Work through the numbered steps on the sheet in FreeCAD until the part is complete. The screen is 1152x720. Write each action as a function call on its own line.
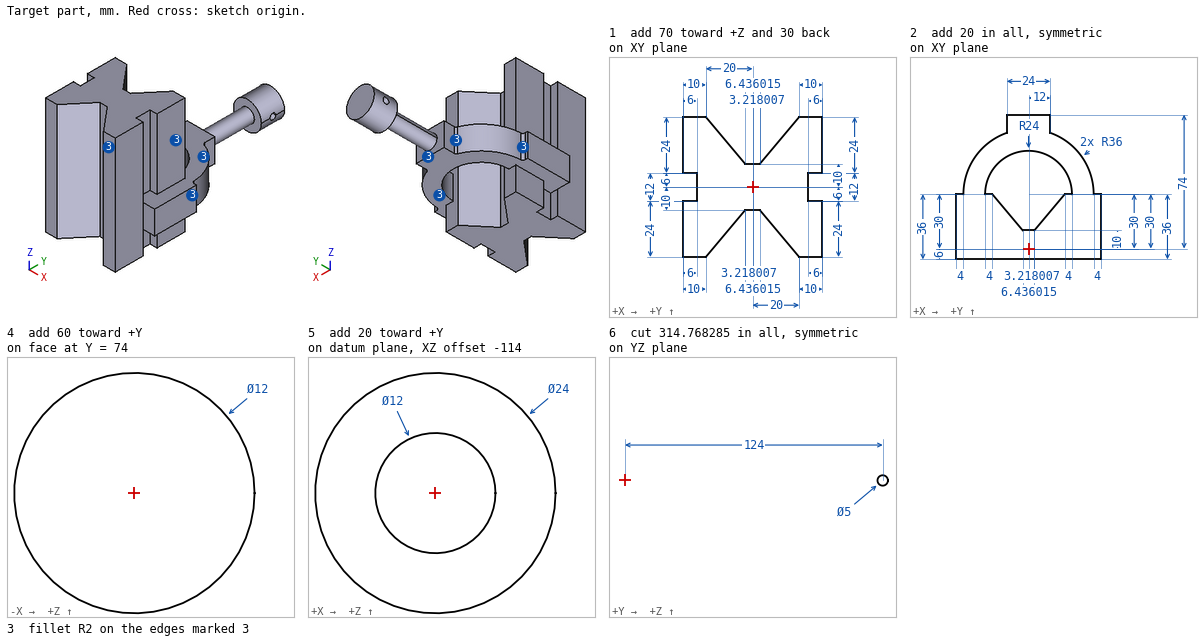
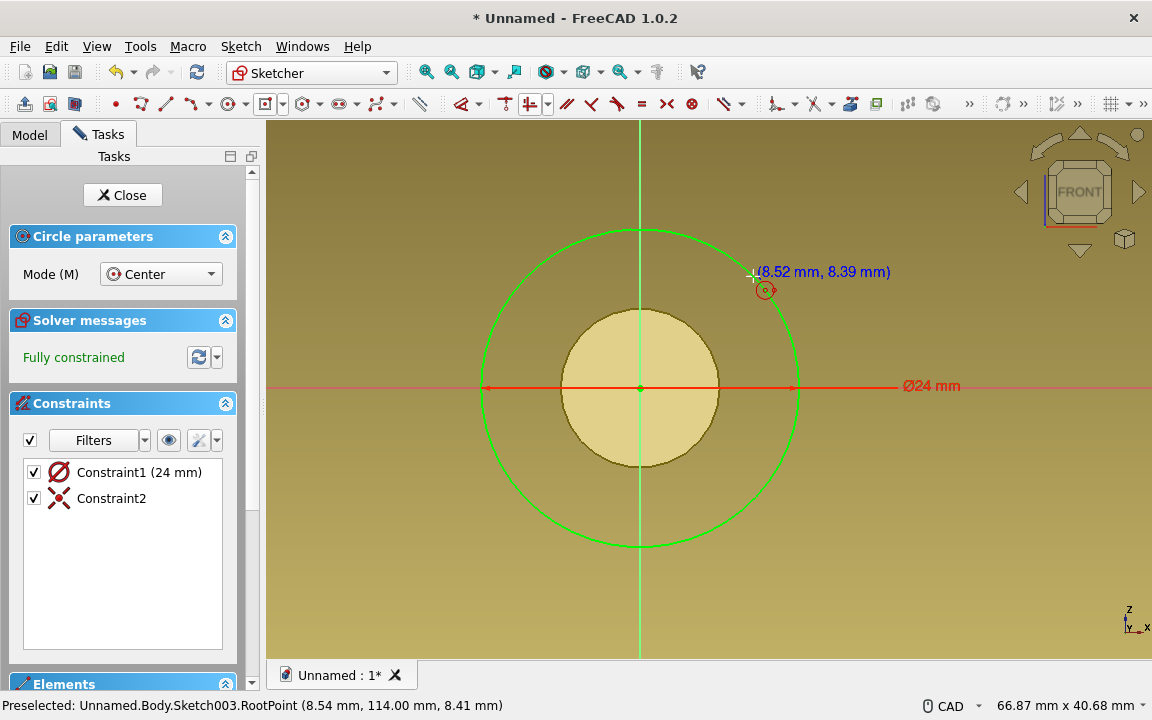
click(640, 388)
move(696, 332)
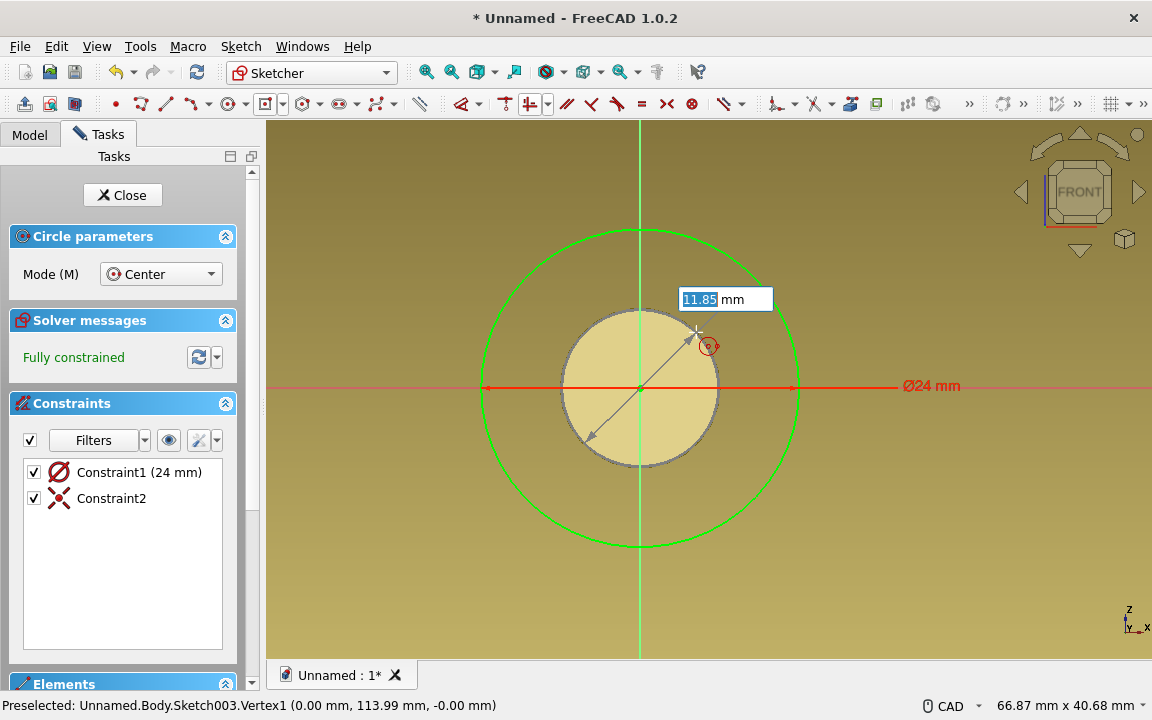
text(12)
key(Return)
key(Escape)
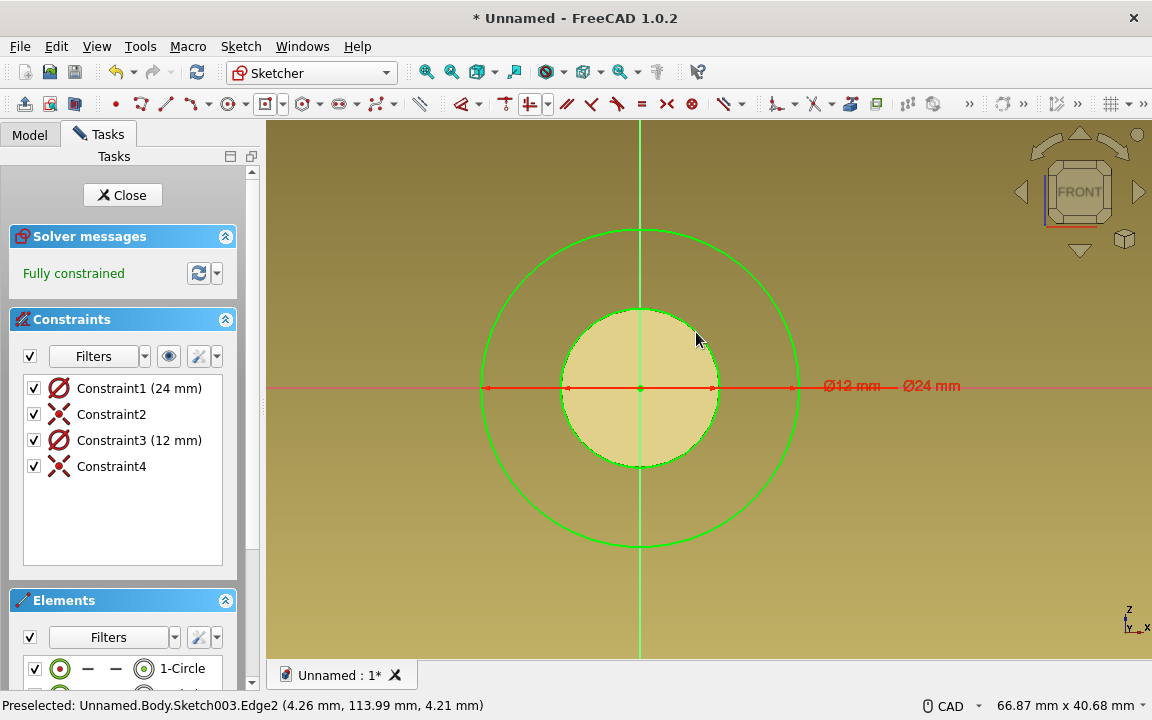
click(123, 195)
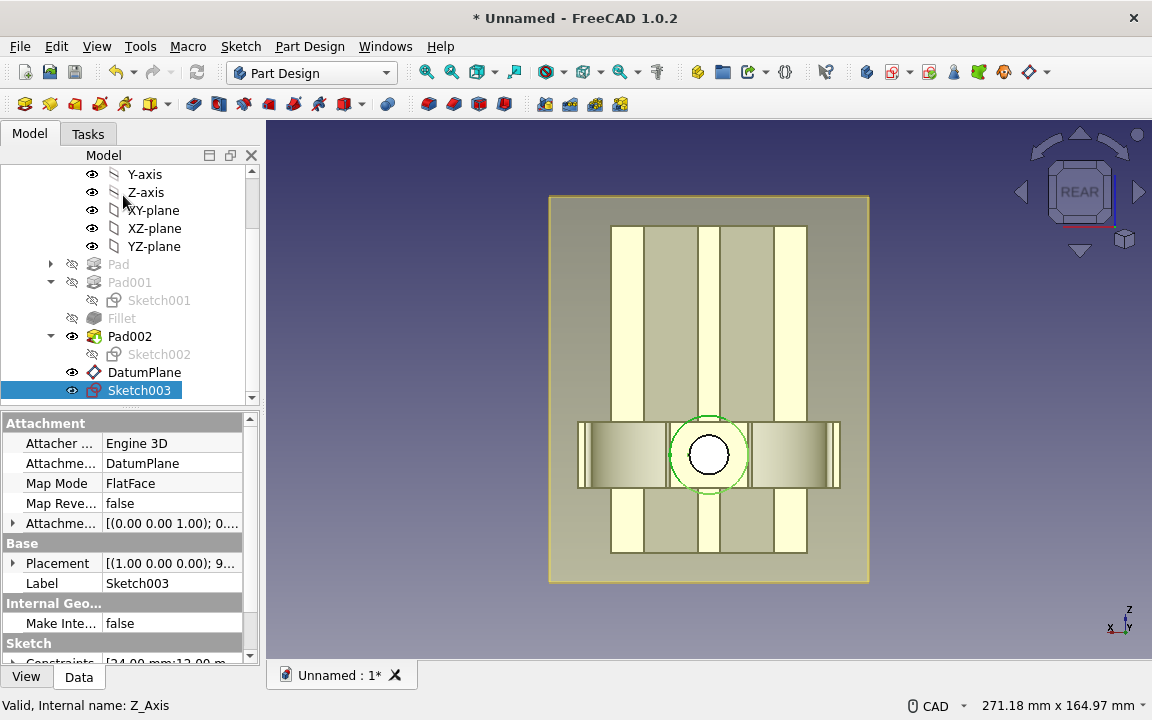
click(25, 104)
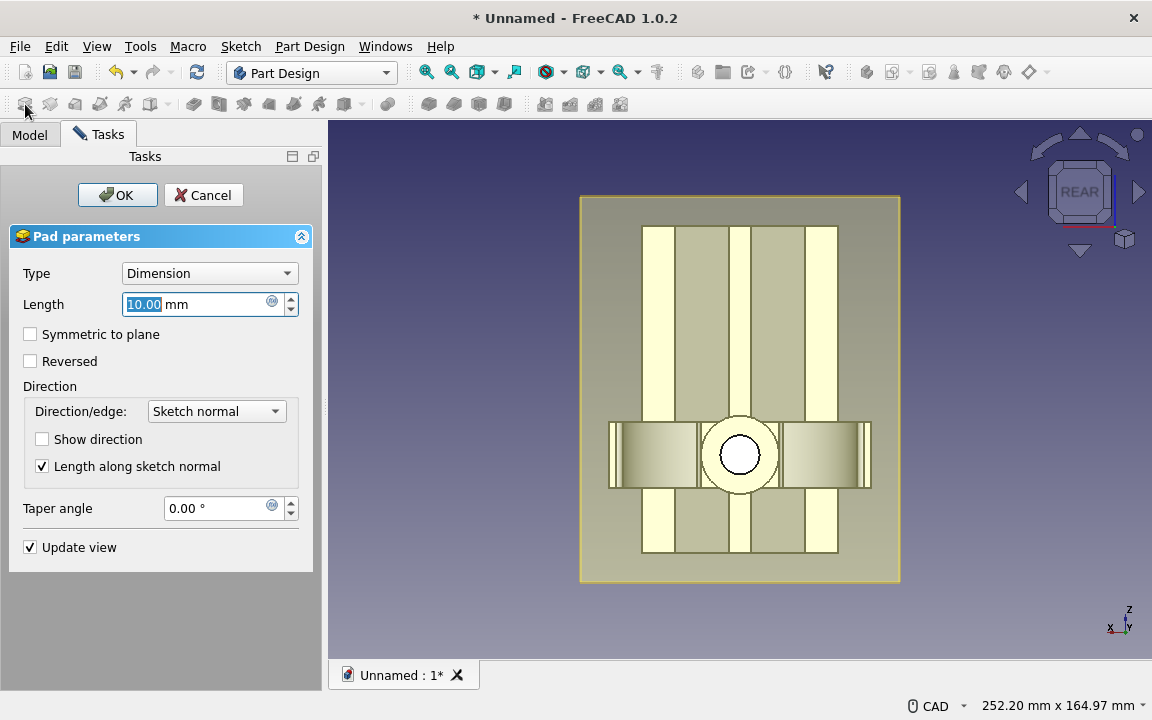
text(20)
key(Tab)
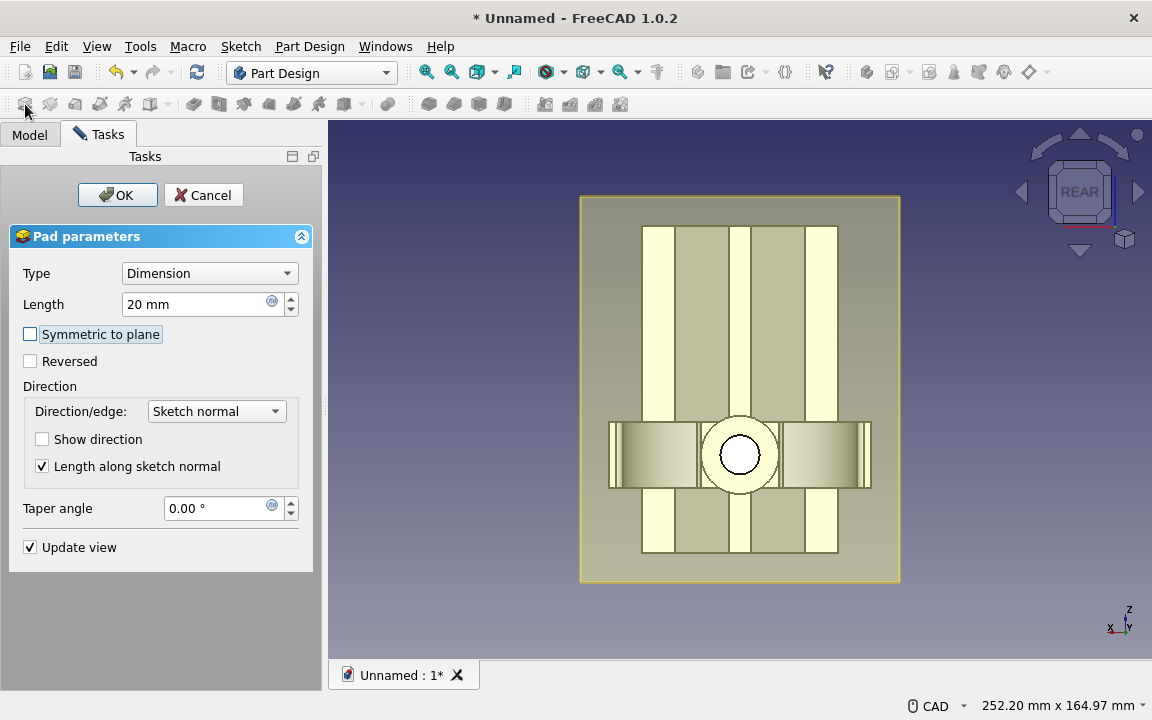
click(31, 361)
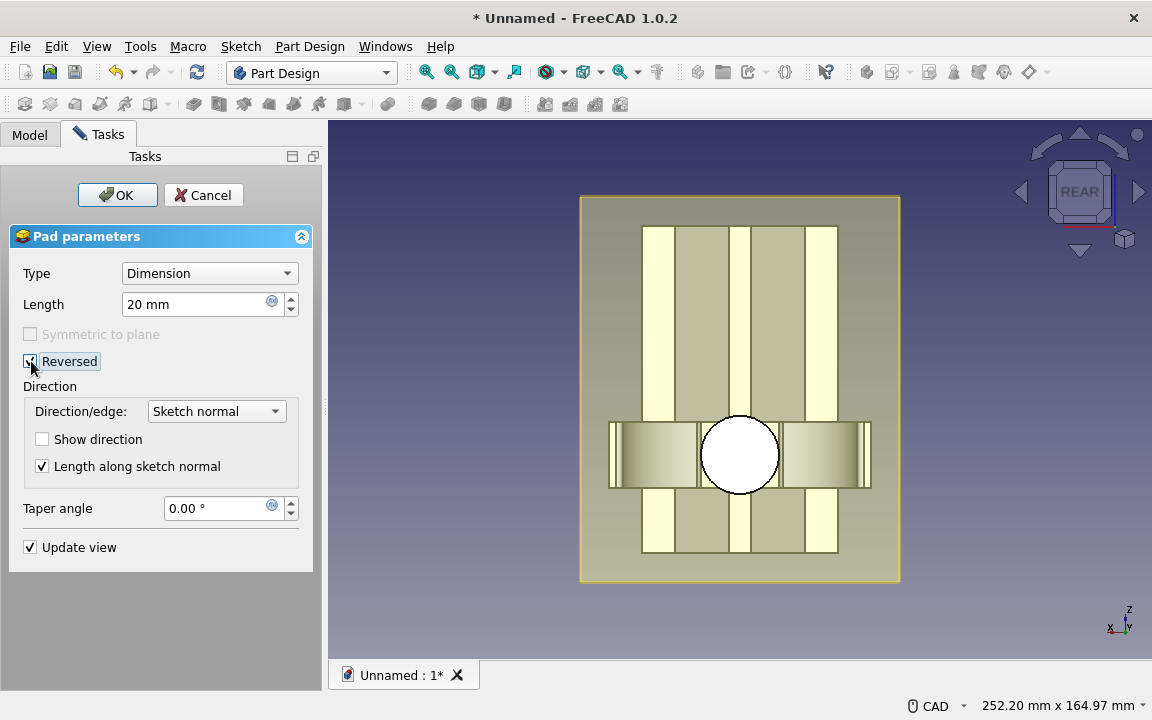
click(118, 195)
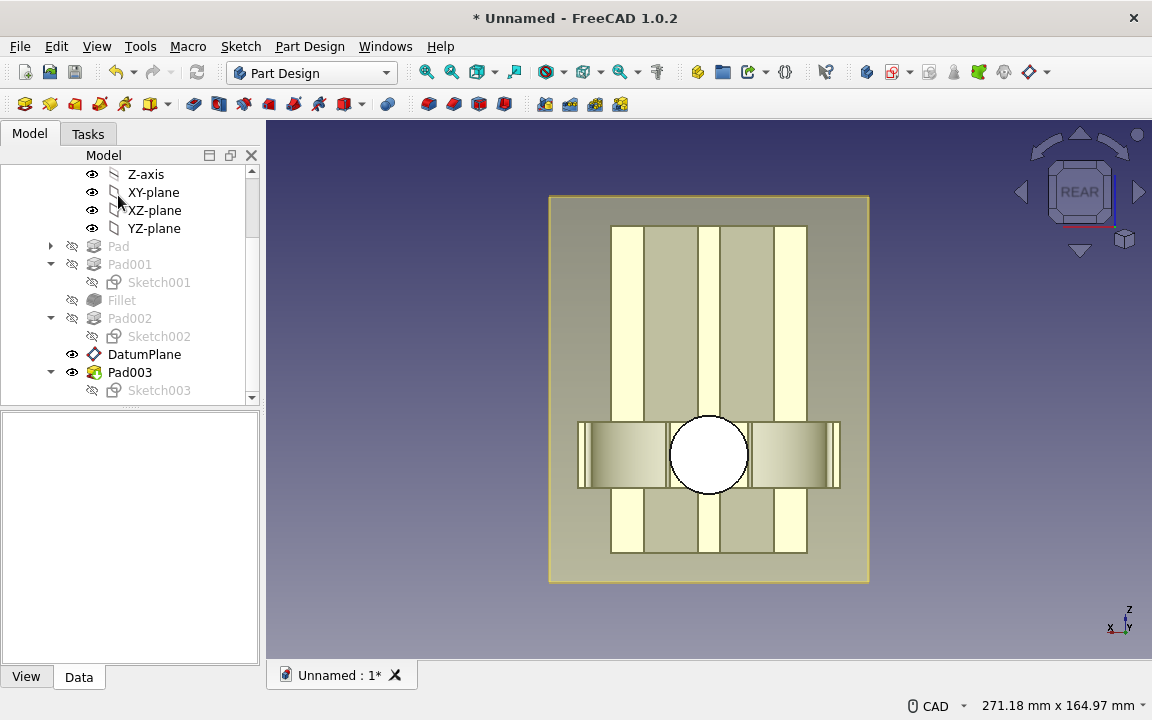
click(117, 354)
key(space)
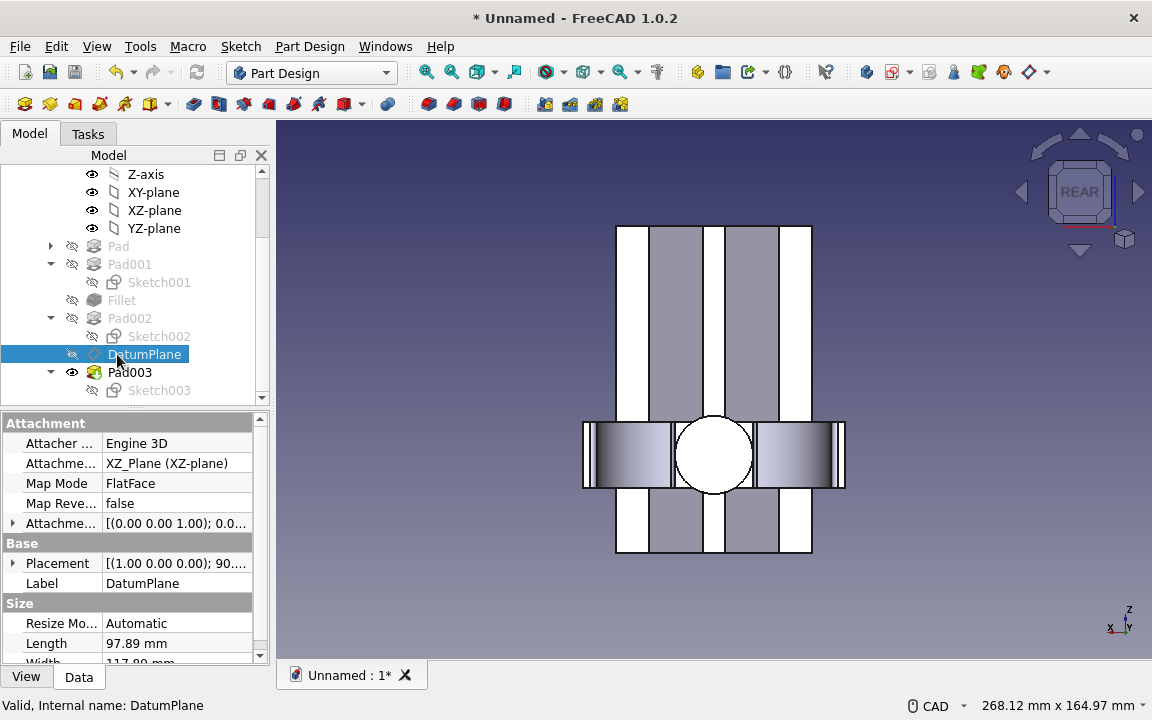
click(316, 619)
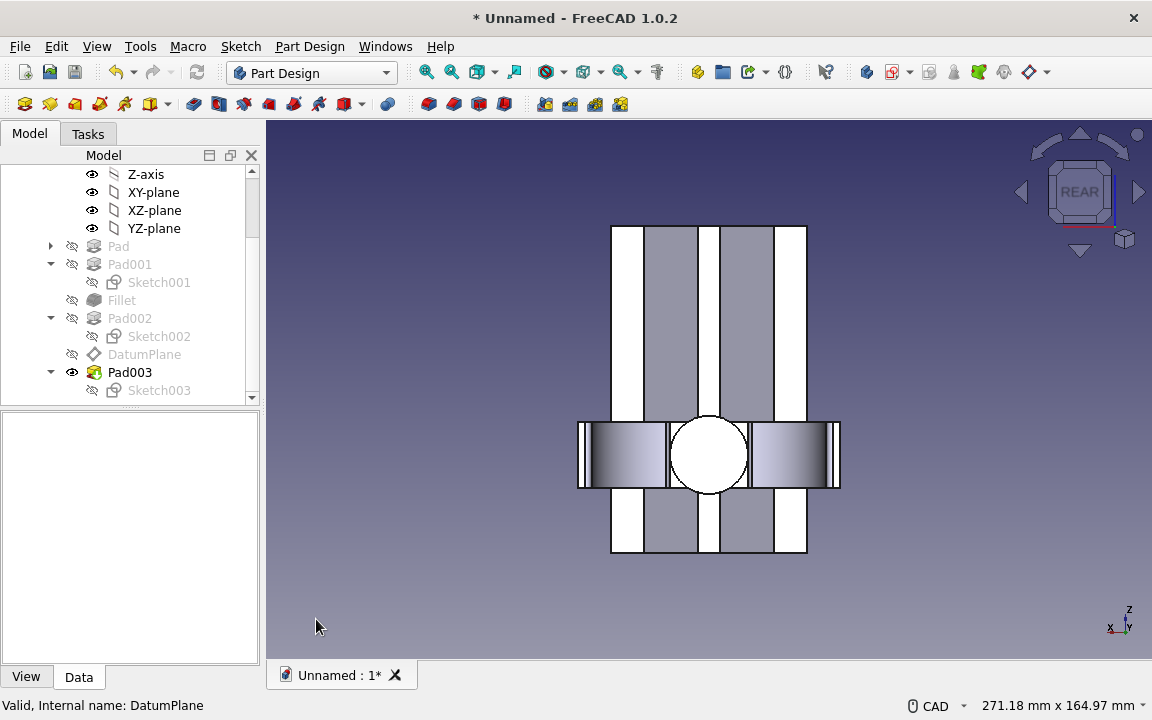
click(892, 72)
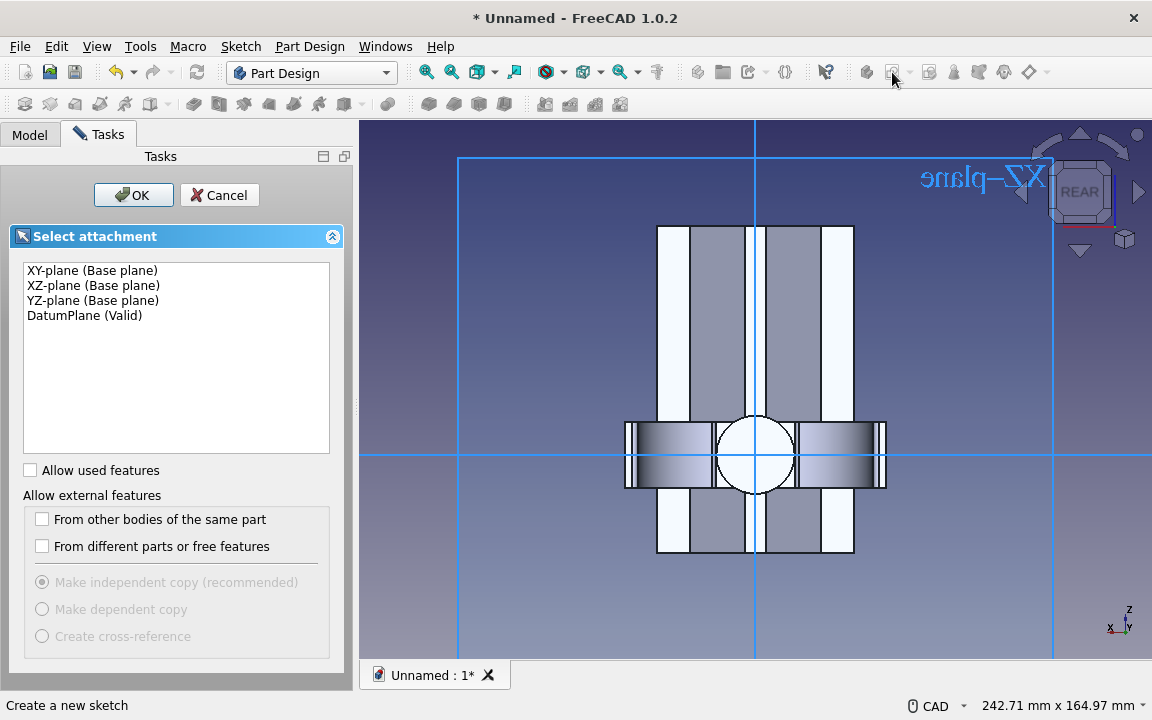
click(84, 300)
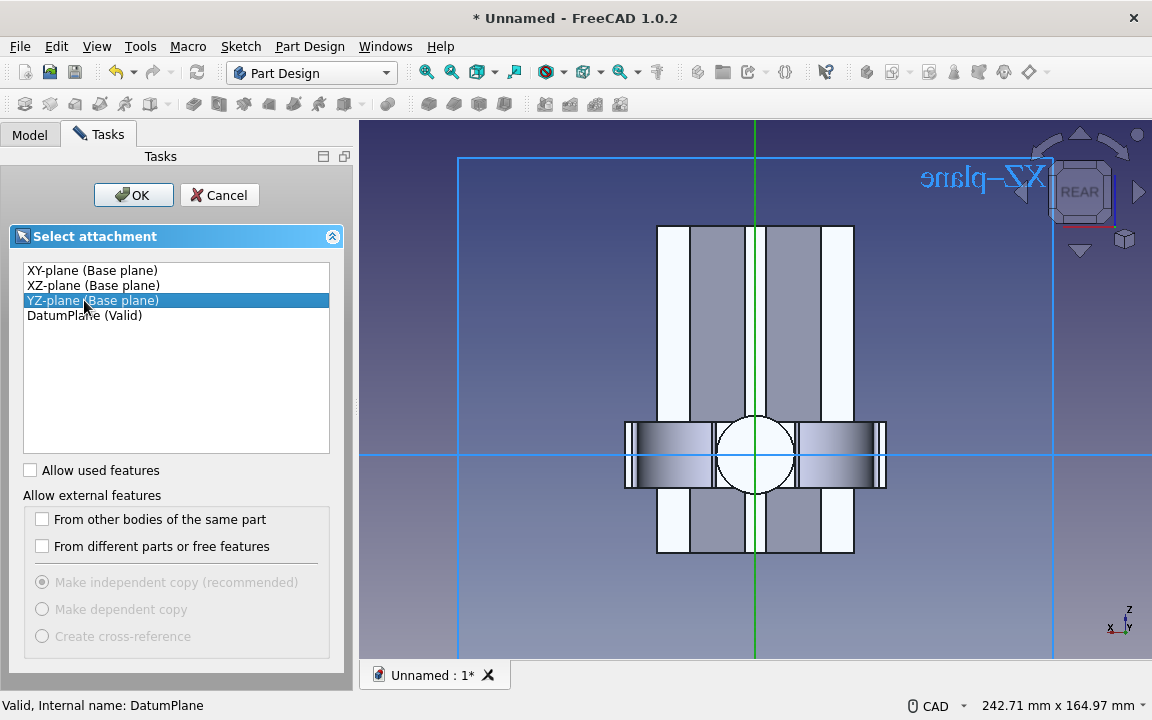
click(134, 195)